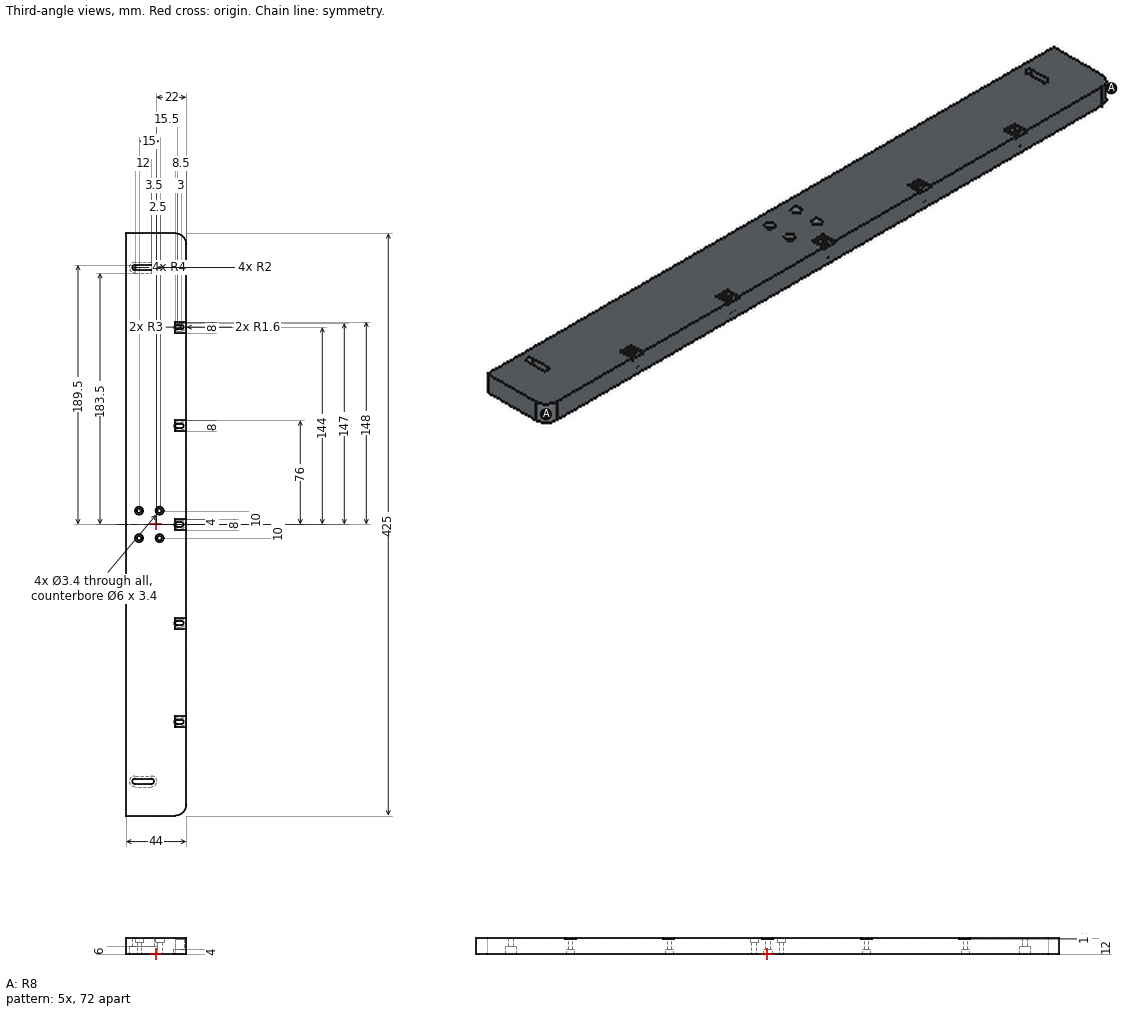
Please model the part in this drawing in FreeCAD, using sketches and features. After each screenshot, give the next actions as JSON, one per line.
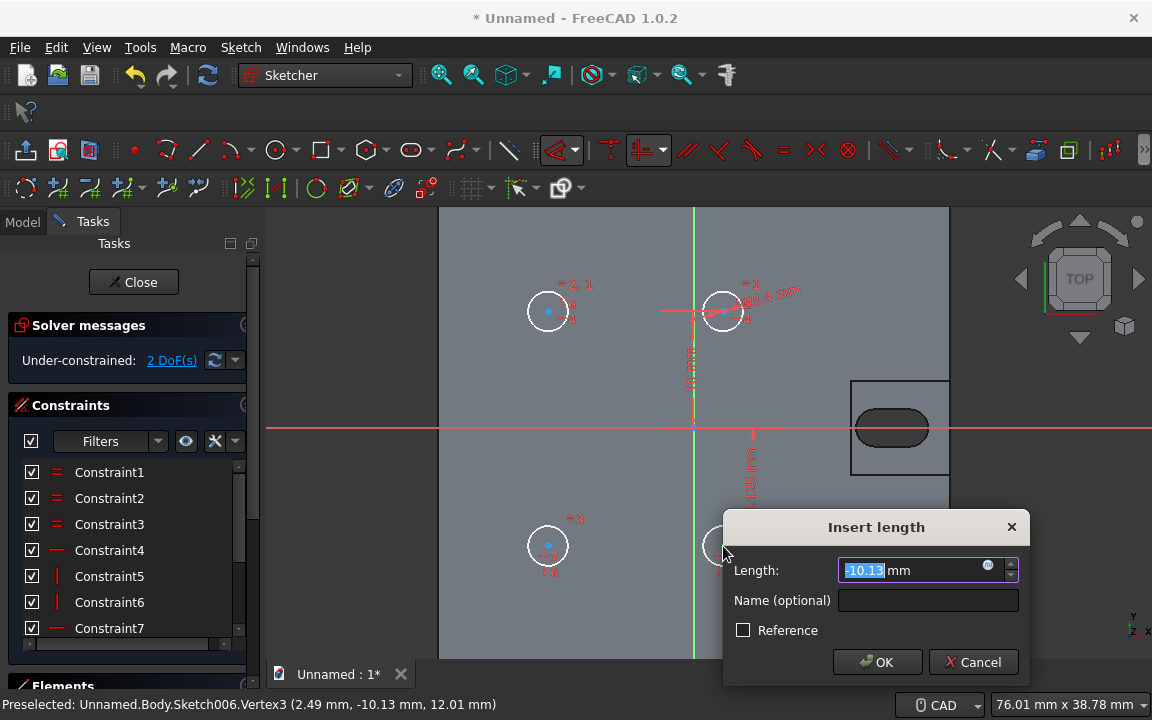
{"action": "type", "text": "-10"}
{"action": "key", "text": "Return"}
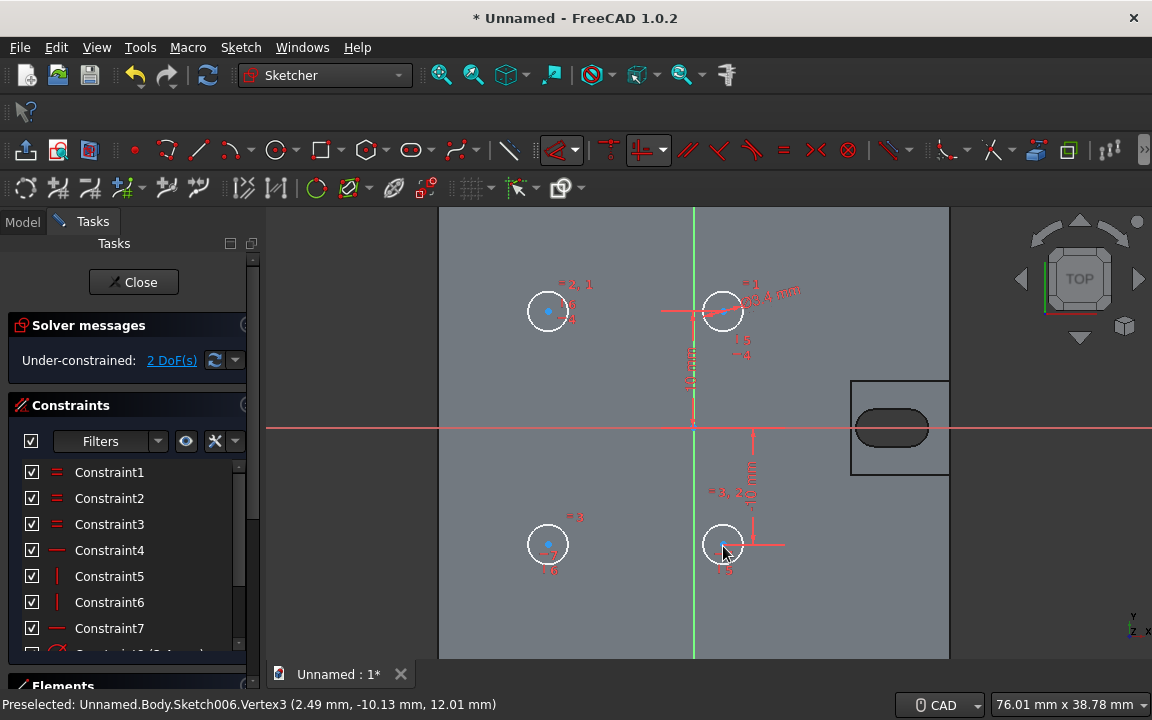
{"action": "scroll", "coordinate": [723, 311], "scroll_direction": "up", "scroll_amount": 2}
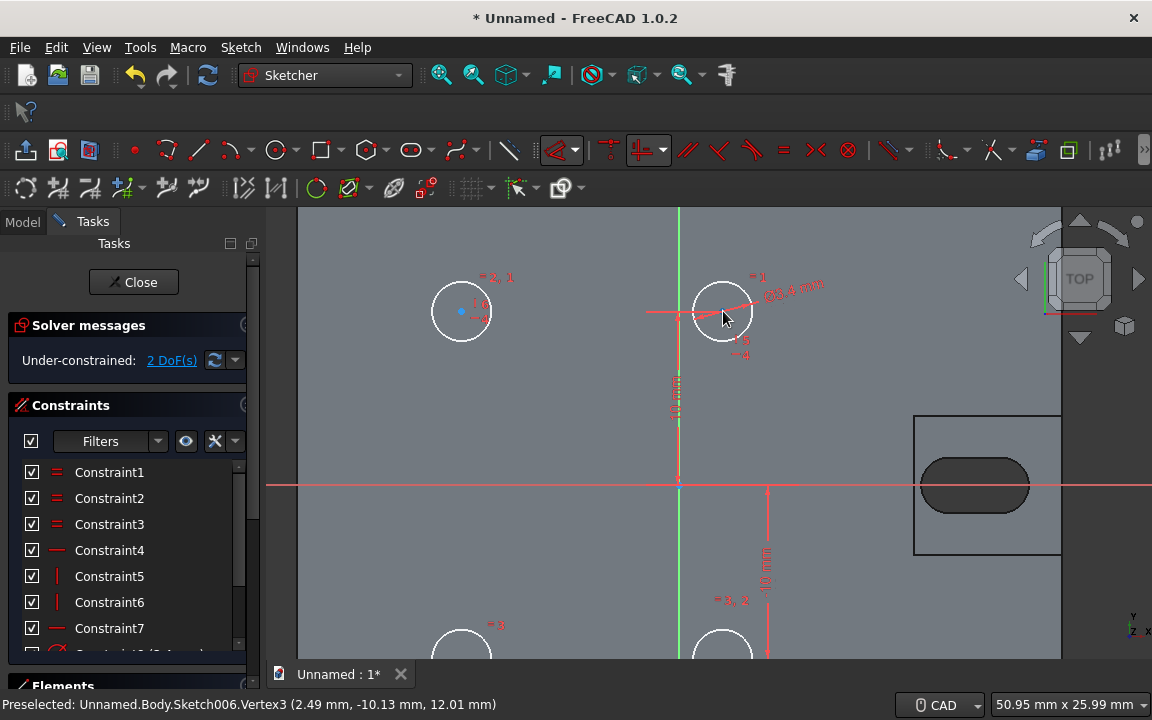
{"action": "left_click", "coordinate": [723, 312]}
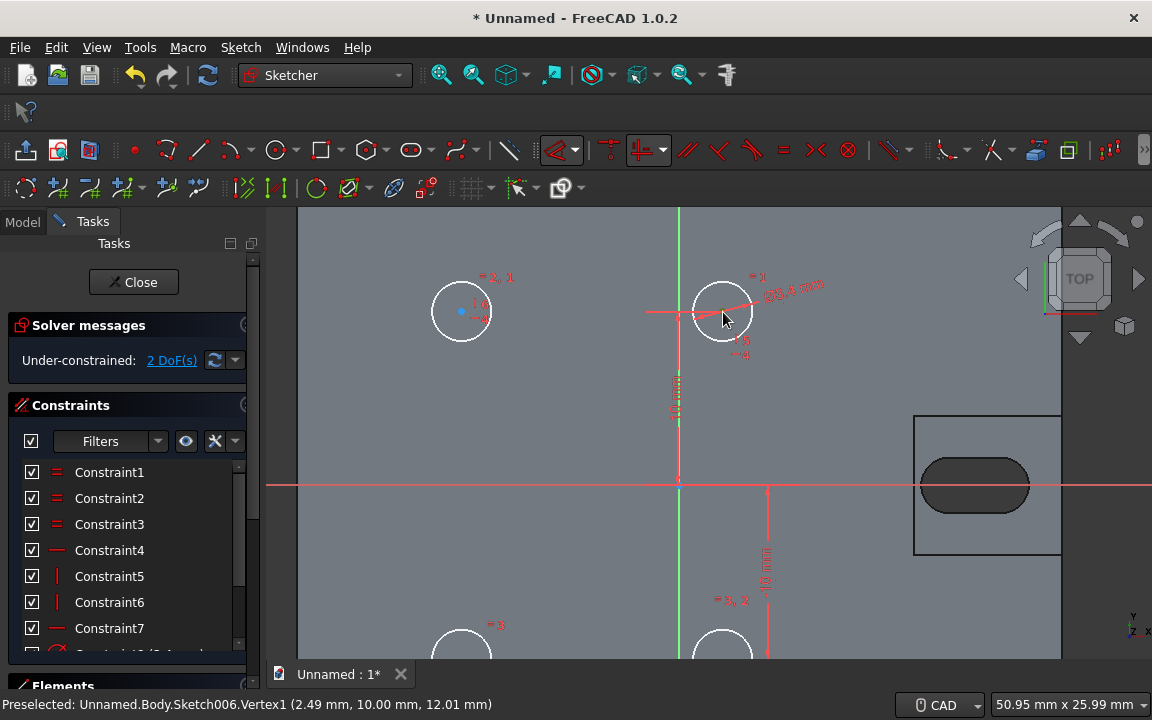
{"action": "key", "text": "l"}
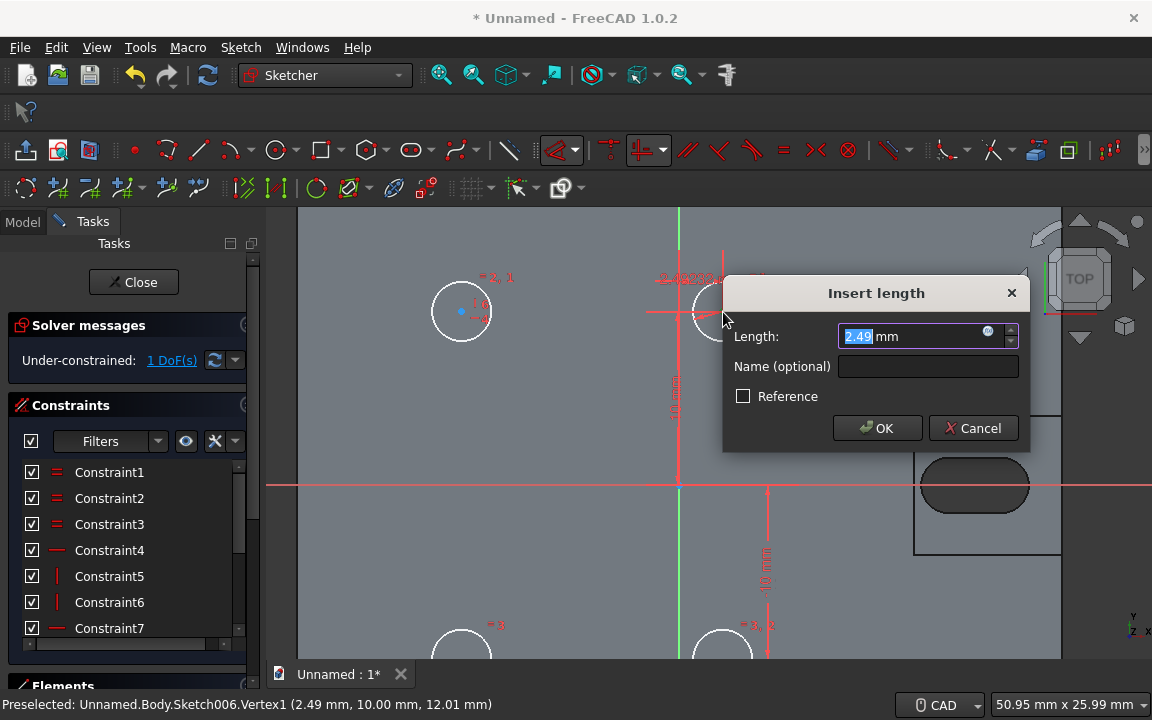
{"action": "type", "text": "2.5"}
{"action": "key", "text": "Return"}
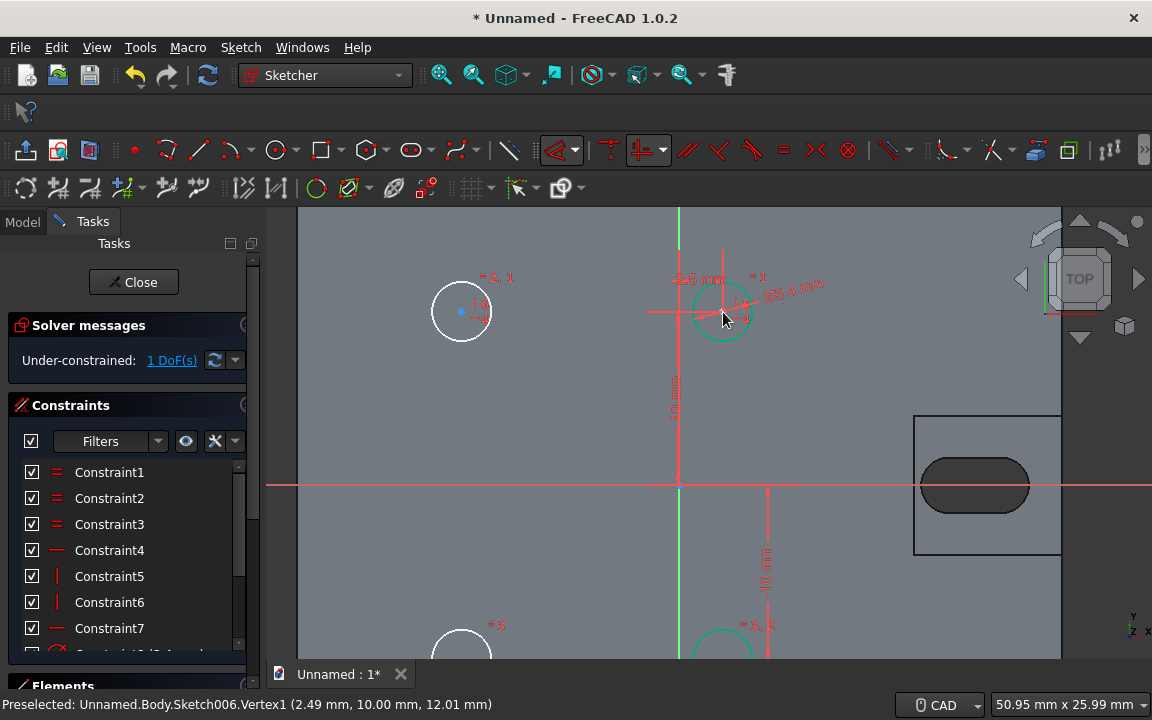
{"action": "left_click", "coordinate": [723, 312]}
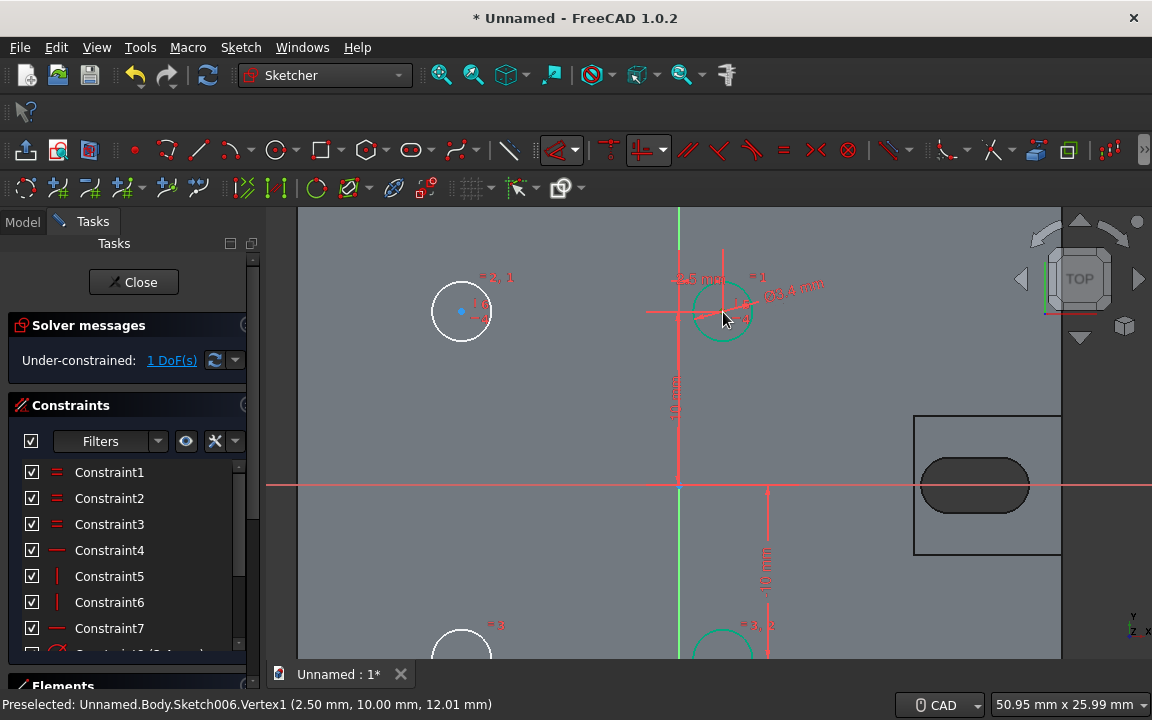
{"action": "left_click", "coordinate": [462, 312]}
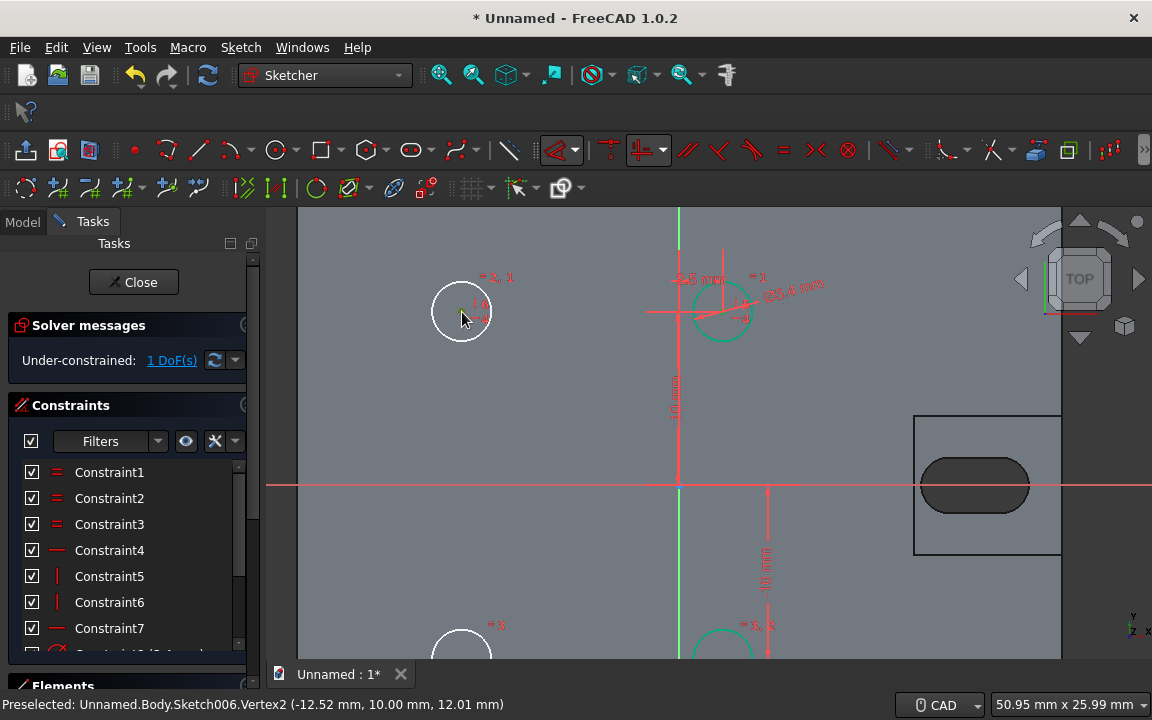
{"action": "key", "text": "l"}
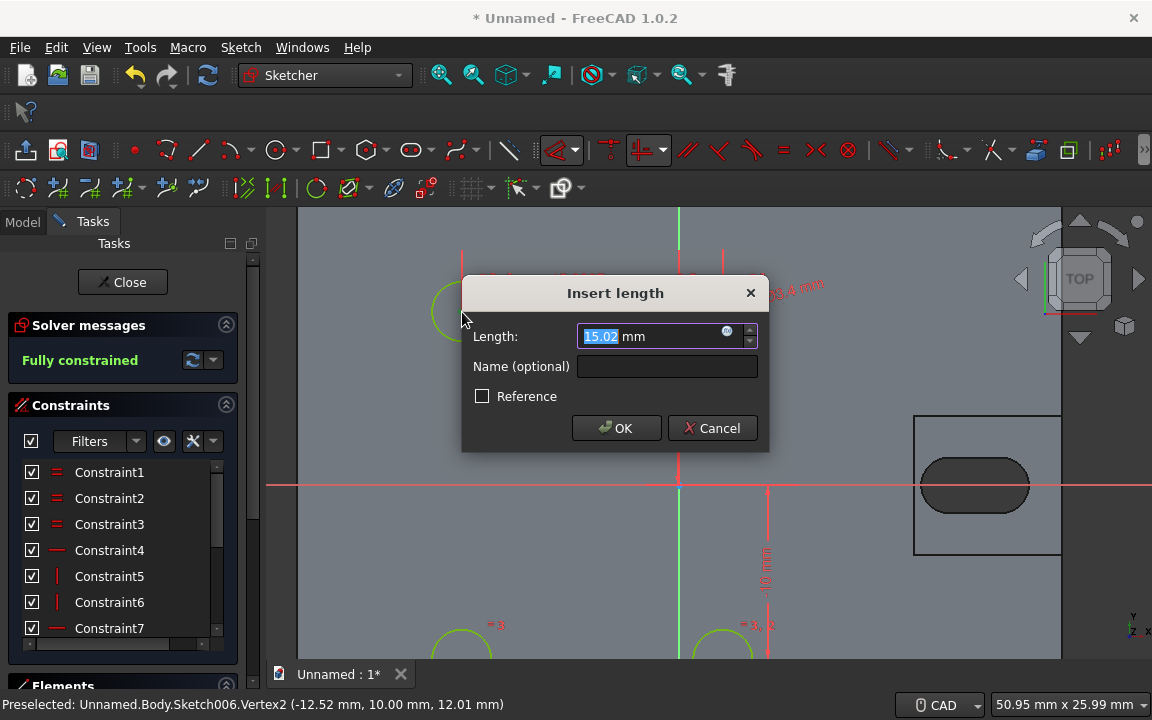
{"action": "type", "text": "15"}
{"action": "key", "text": "Return"}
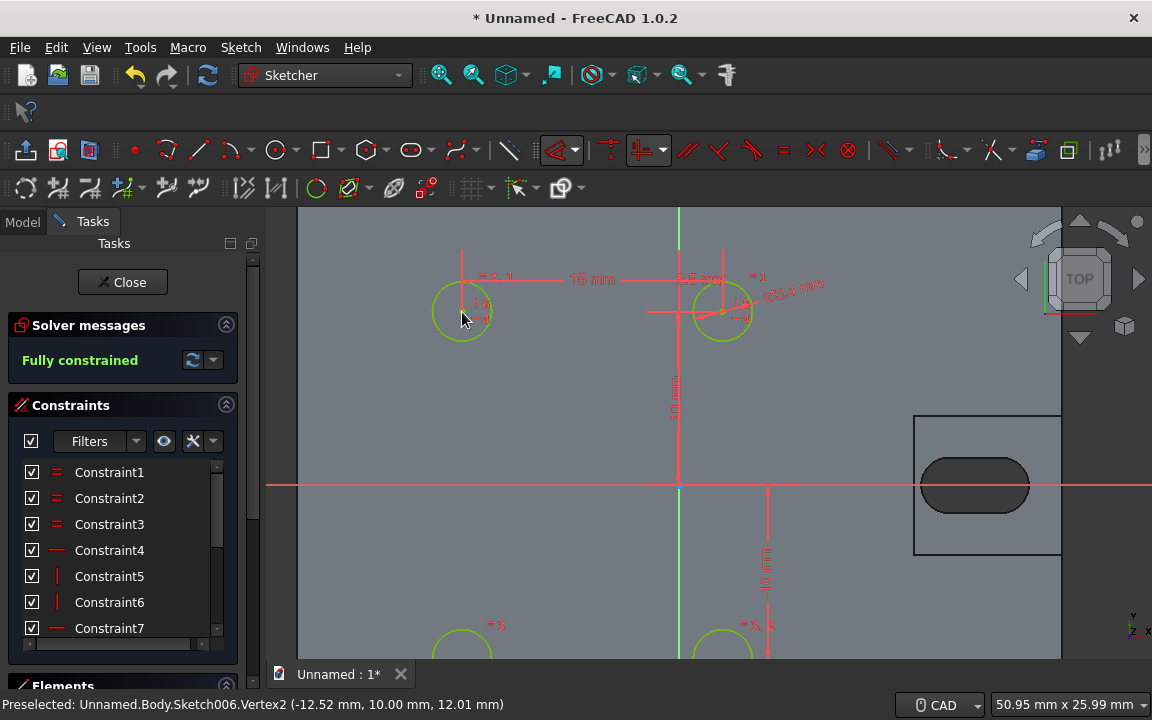
{"action": "left_click", "coordinate": [123, 282]}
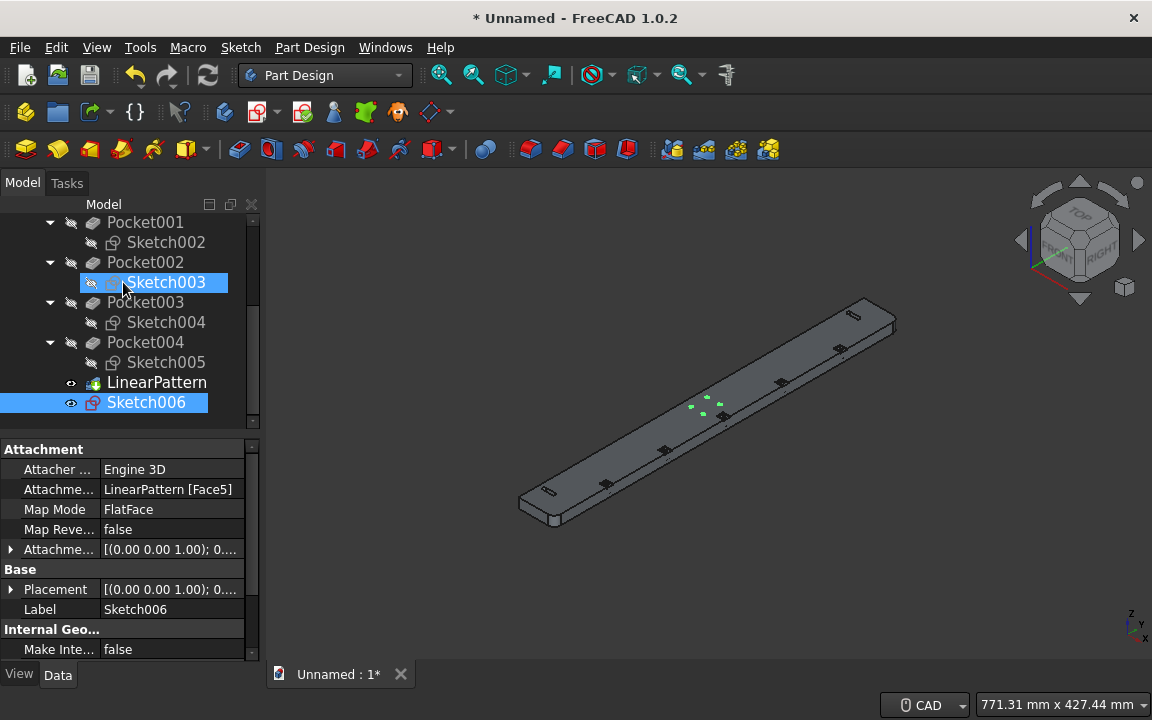
{"action": "left_click", "coordinate": [272, 150]}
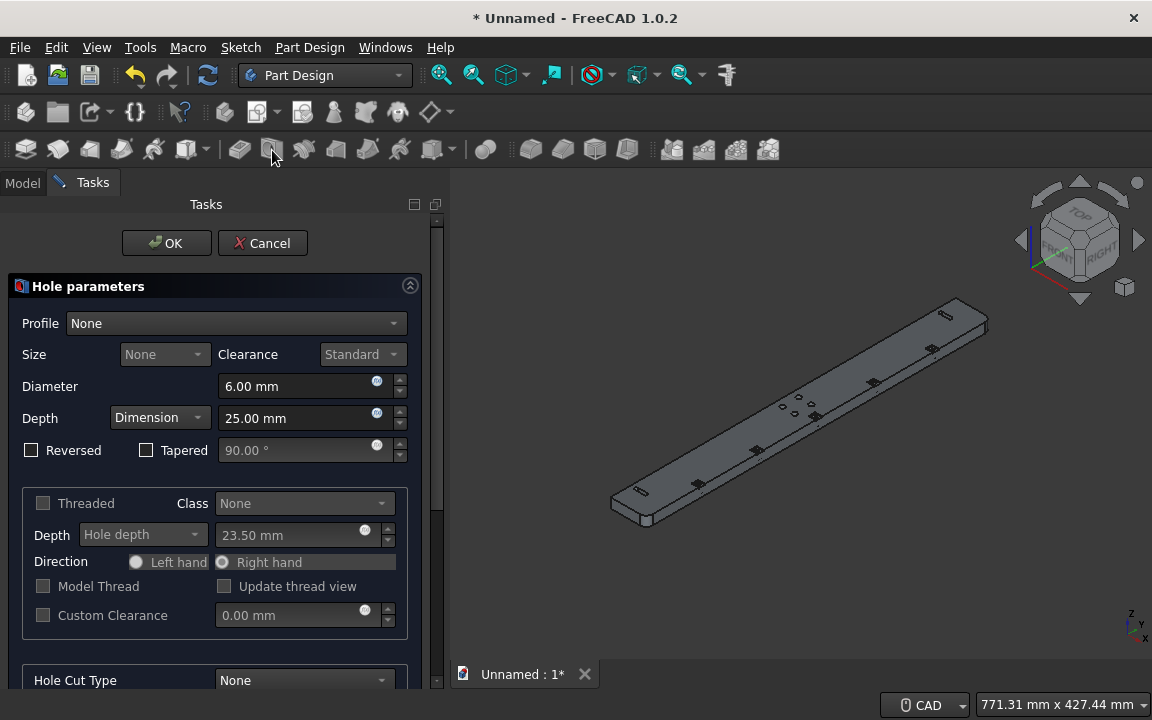
{"action": "triple_click", "coordinate": [305, 386]}